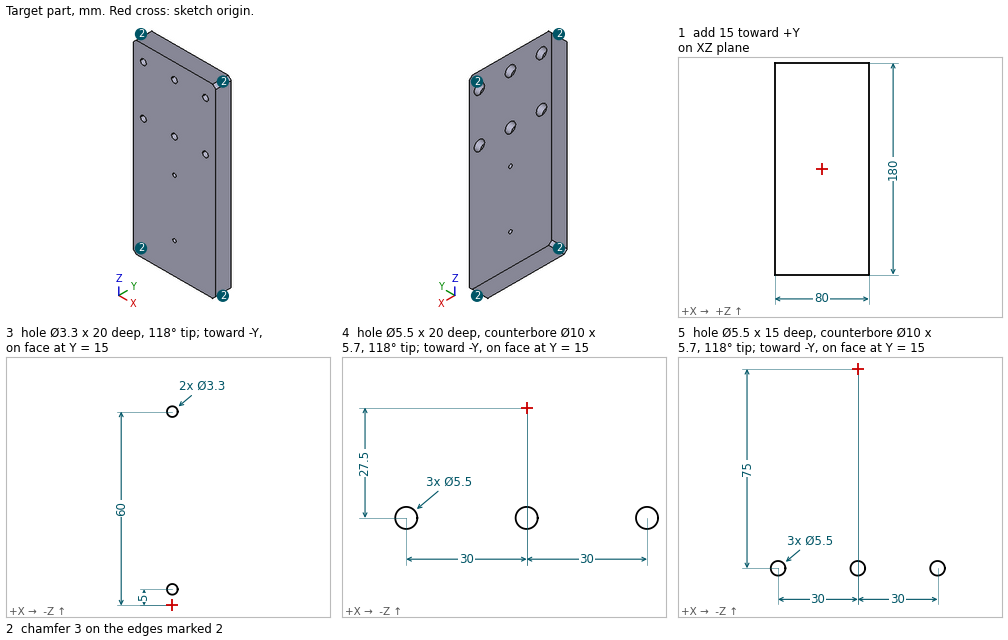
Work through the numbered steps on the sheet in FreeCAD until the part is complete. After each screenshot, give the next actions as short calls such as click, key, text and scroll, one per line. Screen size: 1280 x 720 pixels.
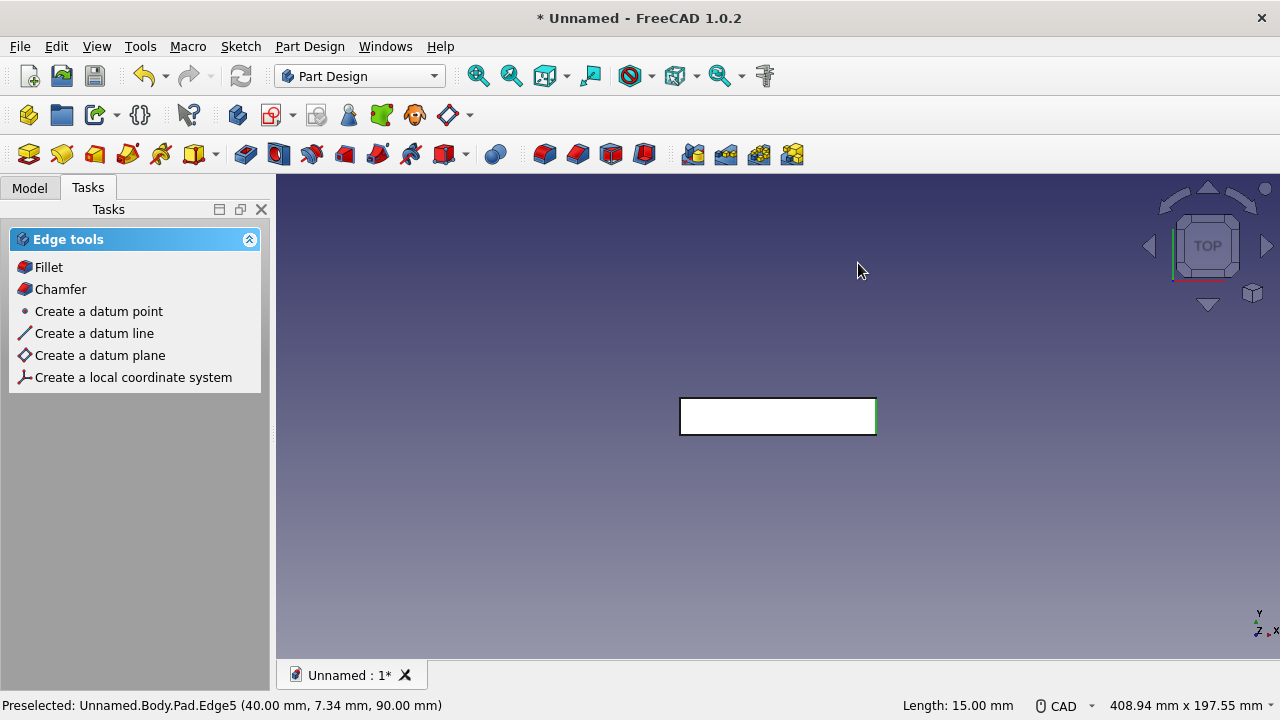
click(479, 76)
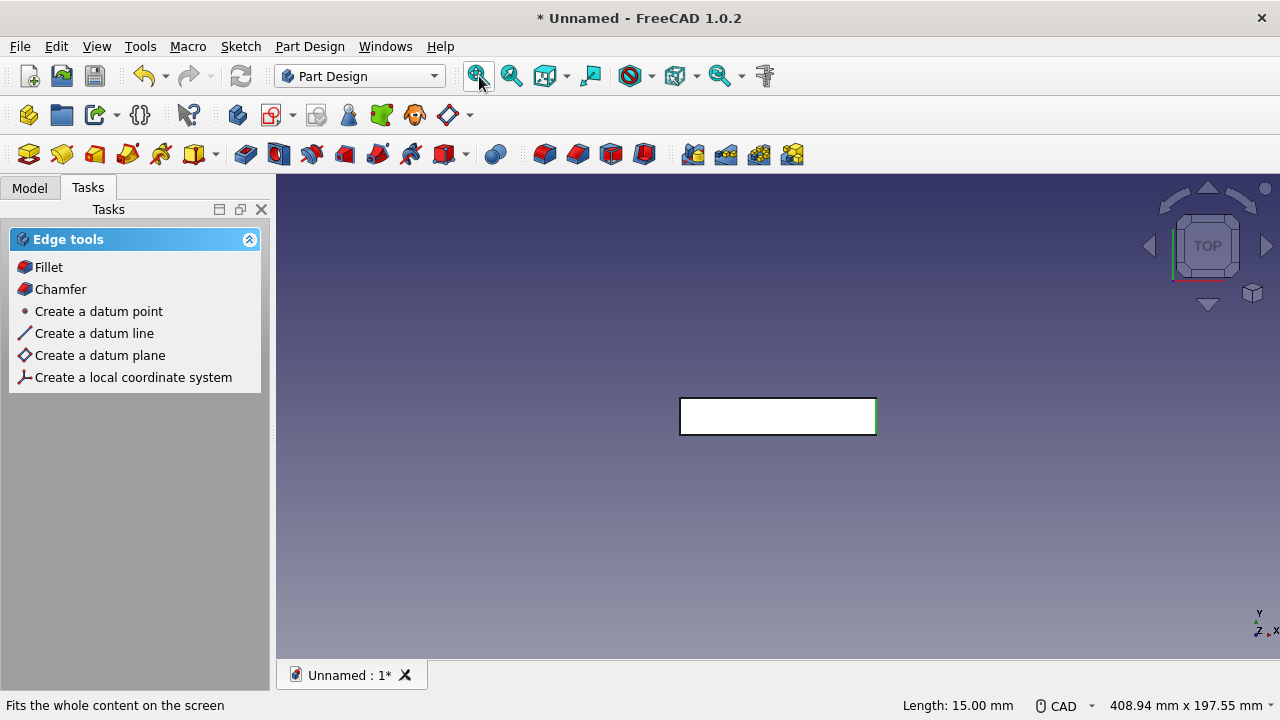
click(680, 415, ctrl)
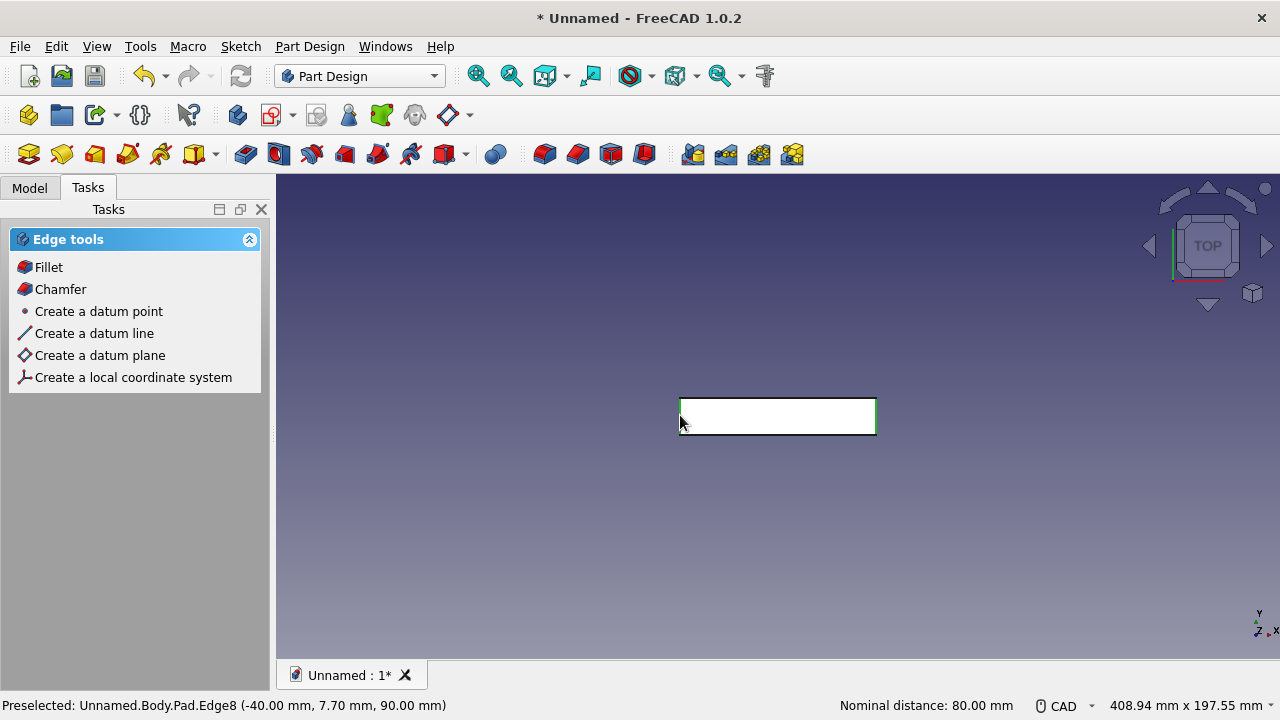
key(1)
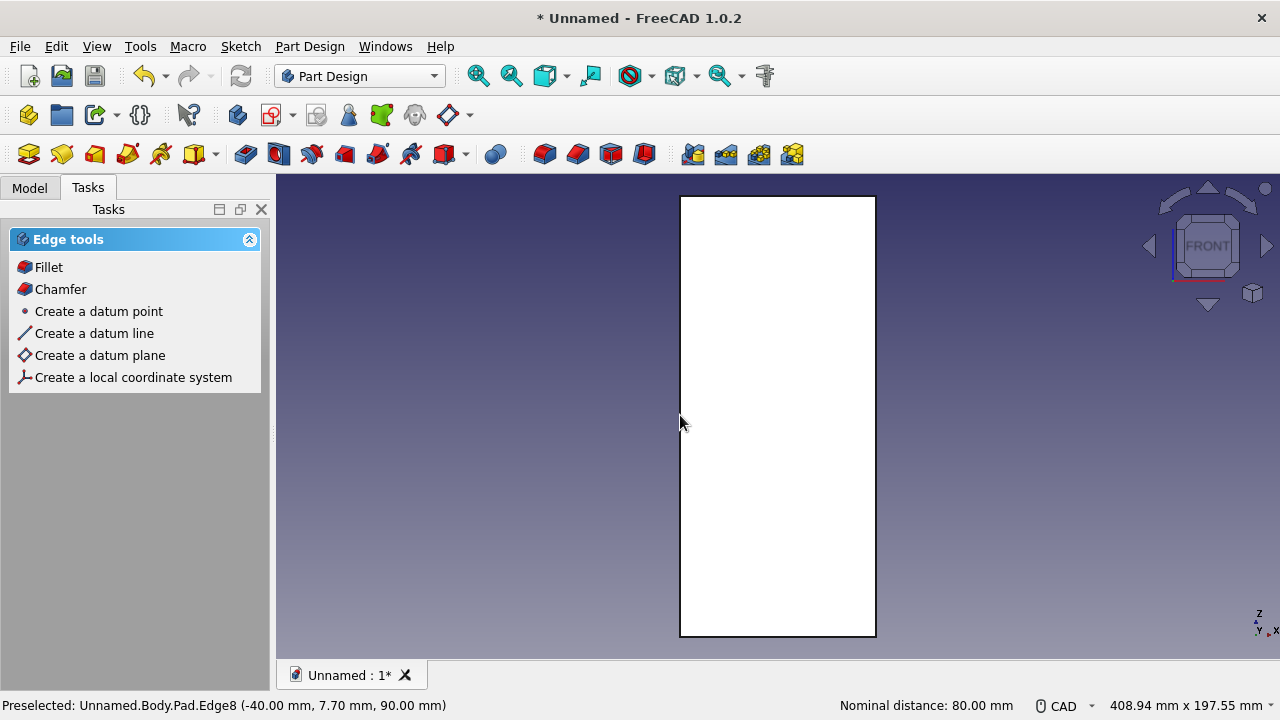
key(3)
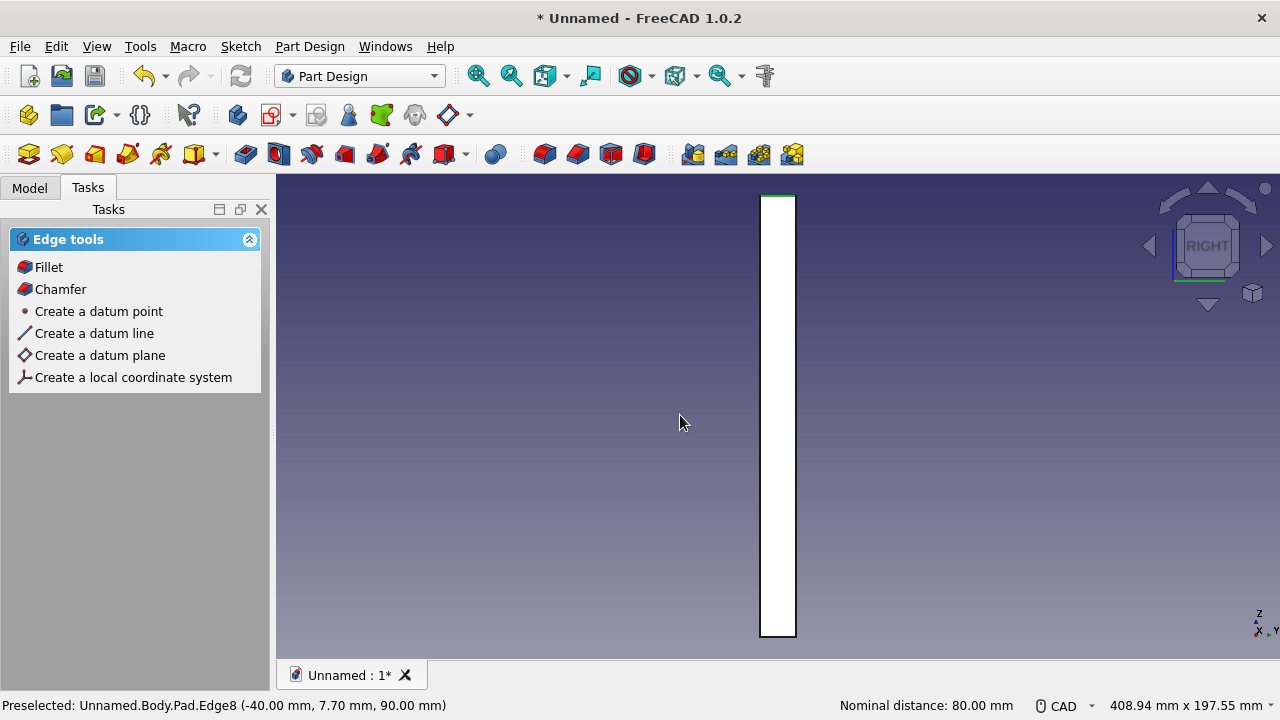
key(5)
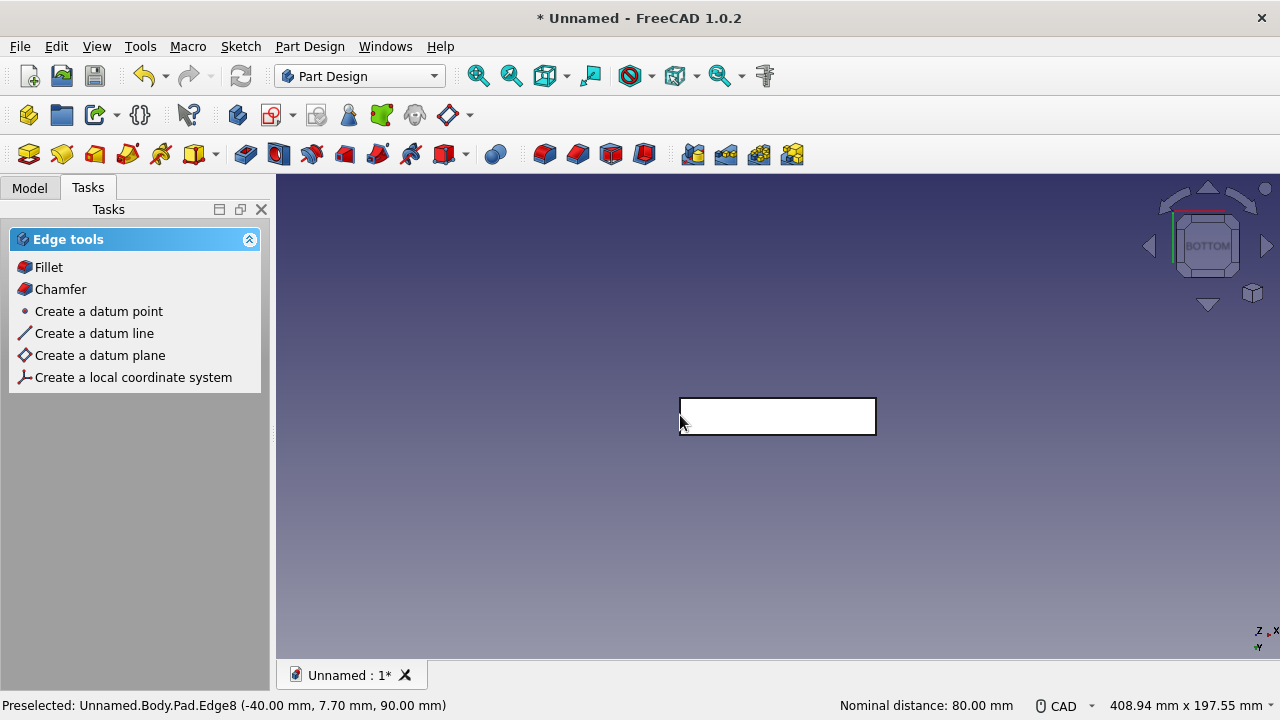
click(479, 76)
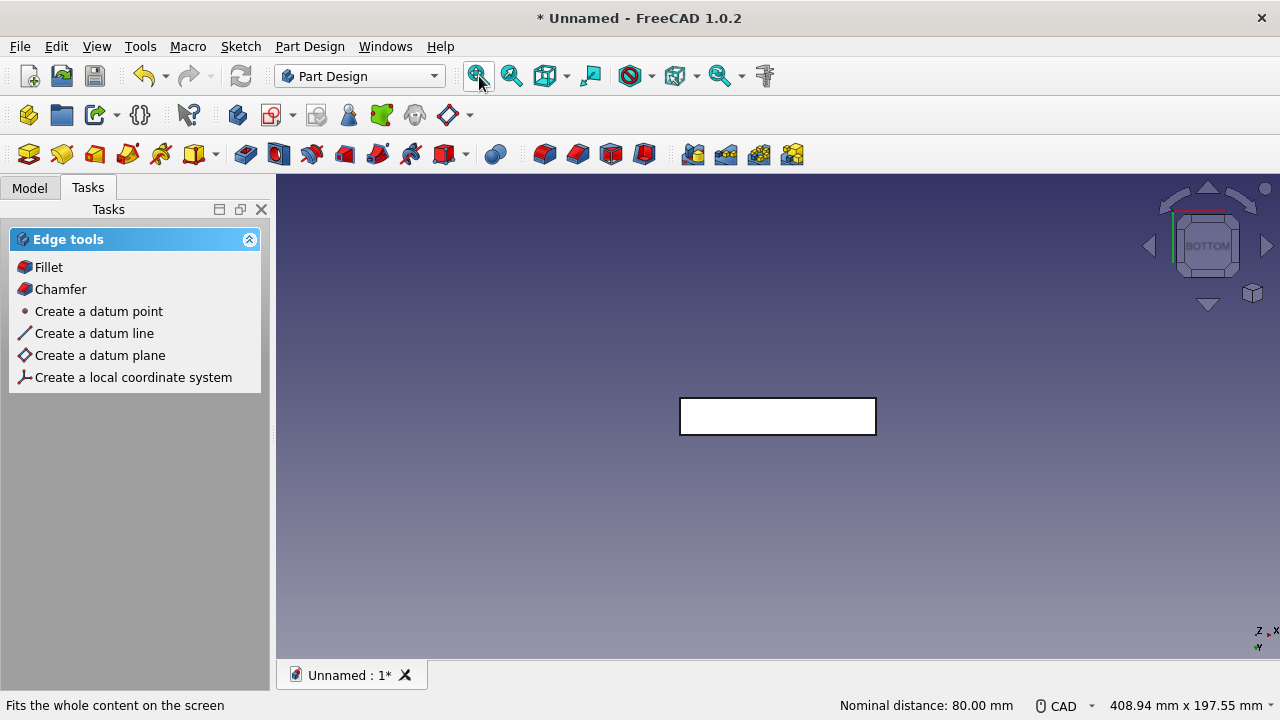
click(680, 415, ctrl)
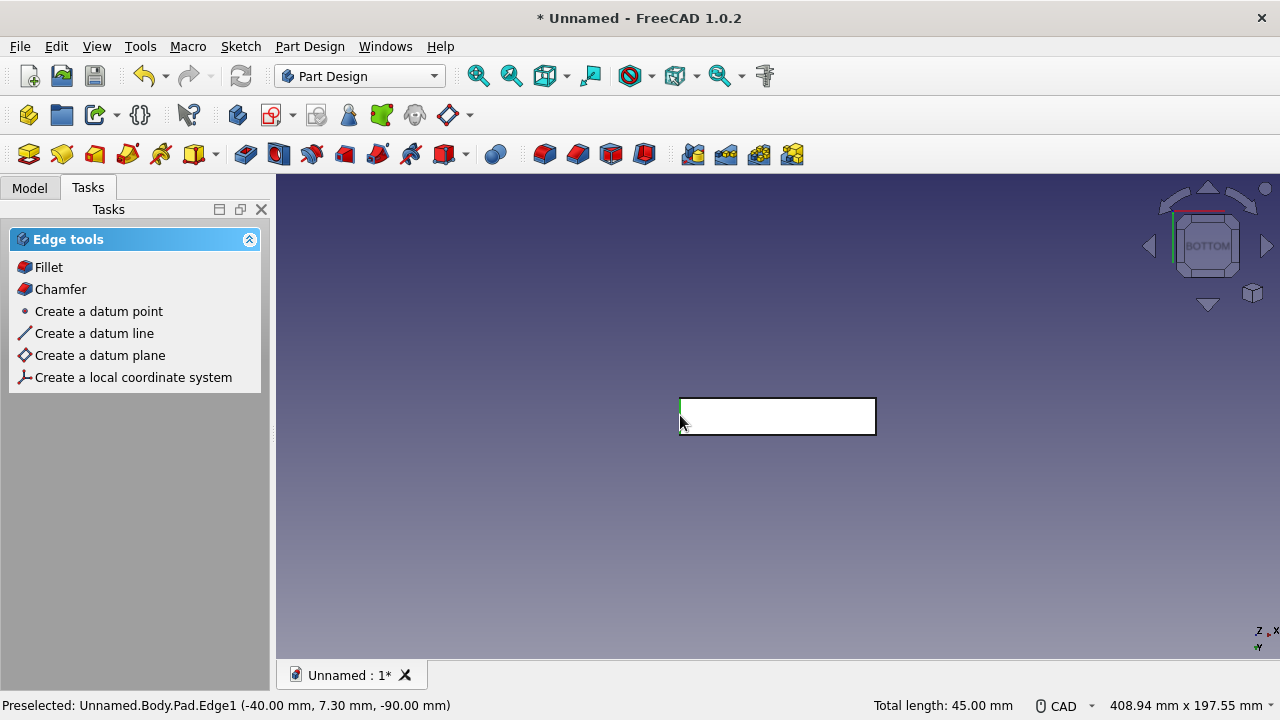
click(876, 415, ctrl)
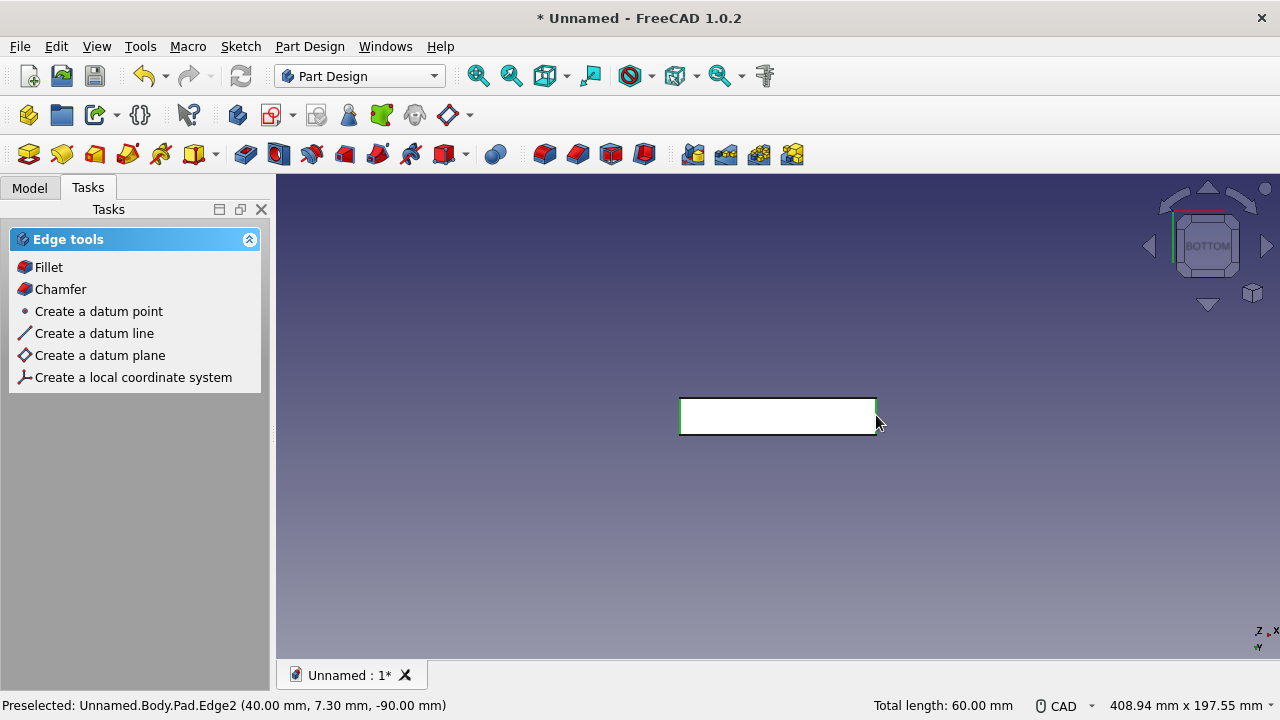
click(578, 154)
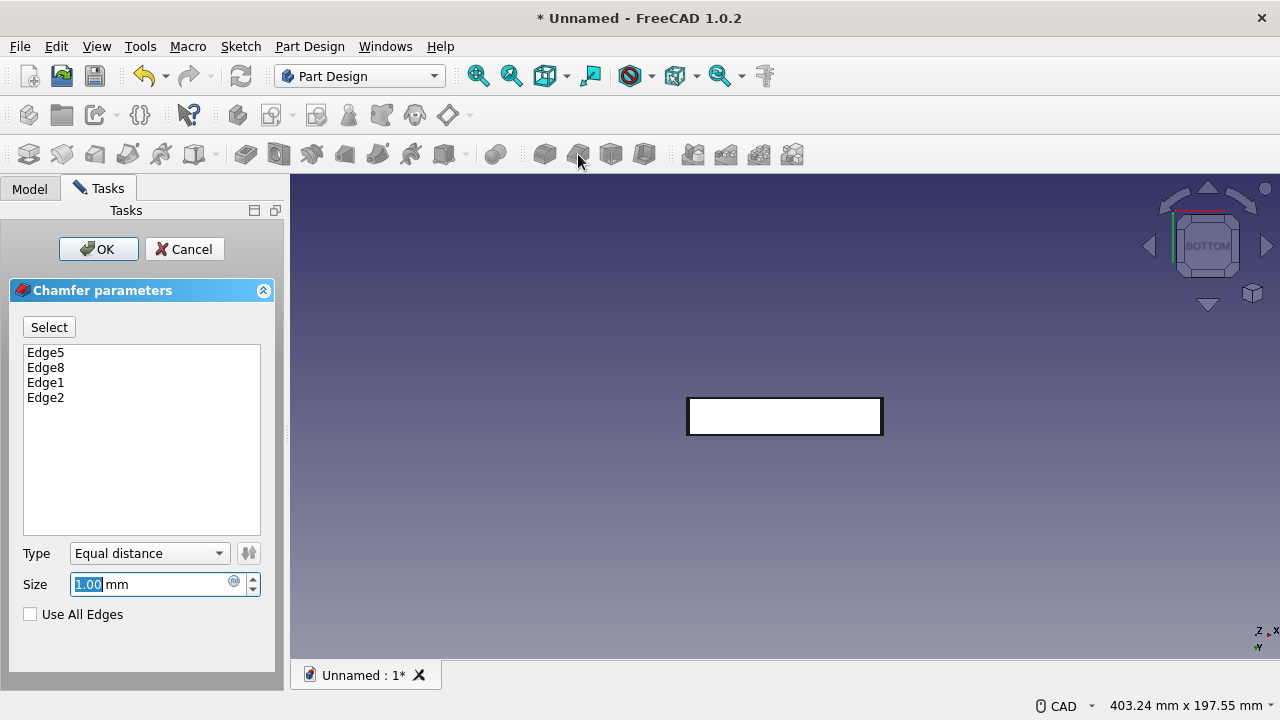
text(3)
key(Tab)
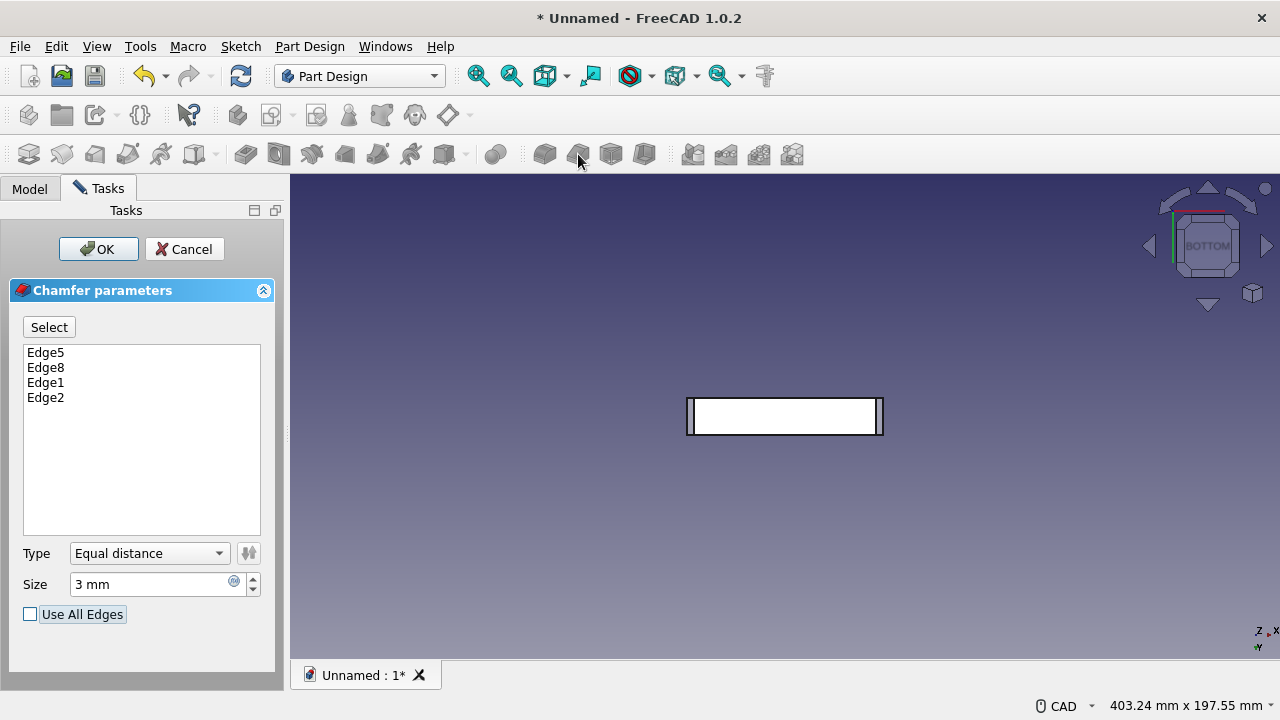
click(99, 249)